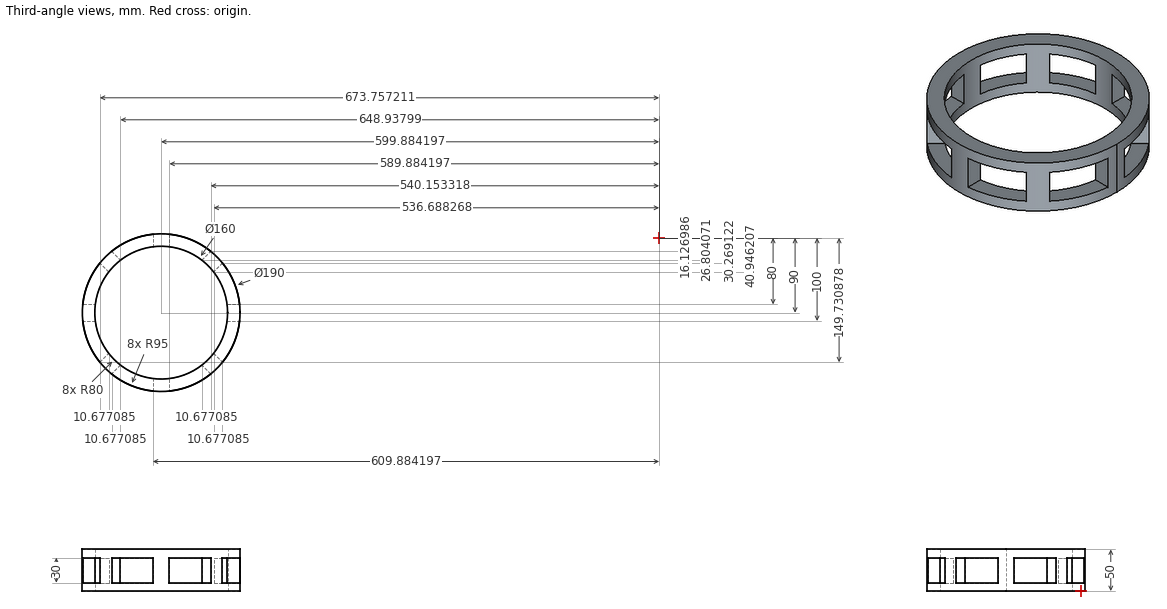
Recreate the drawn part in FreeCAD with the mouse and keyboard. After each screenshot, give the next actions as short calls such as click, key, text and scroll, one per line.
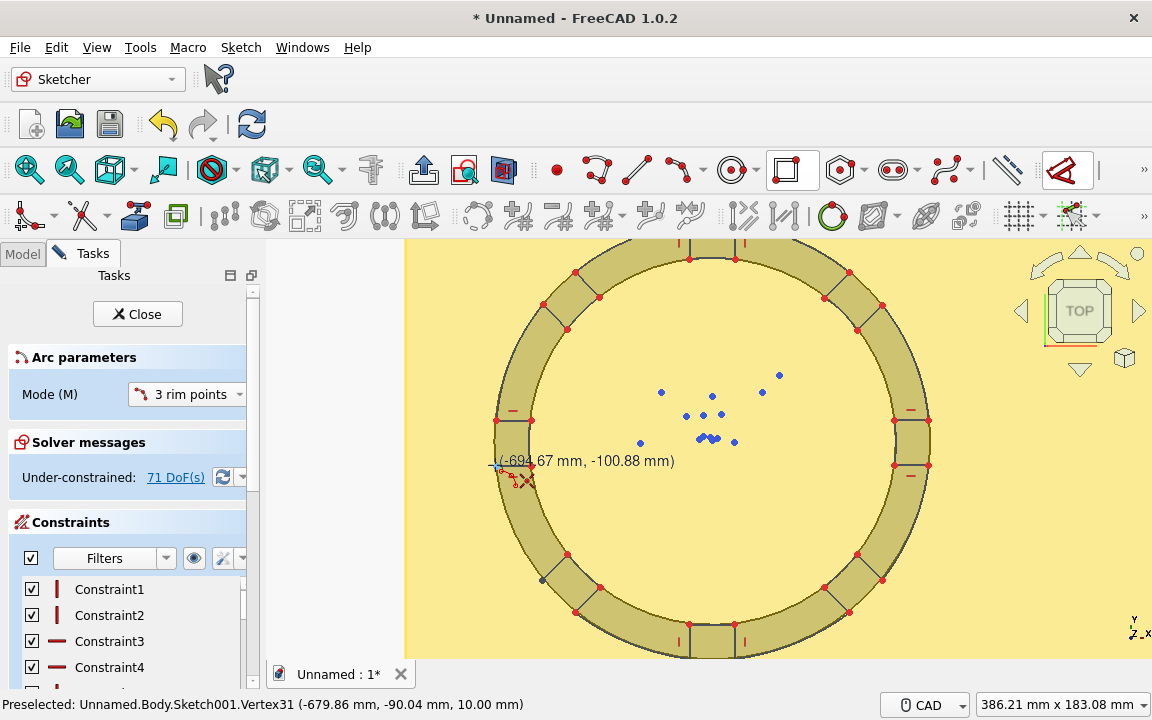
click(496, 466)
click(542, 580)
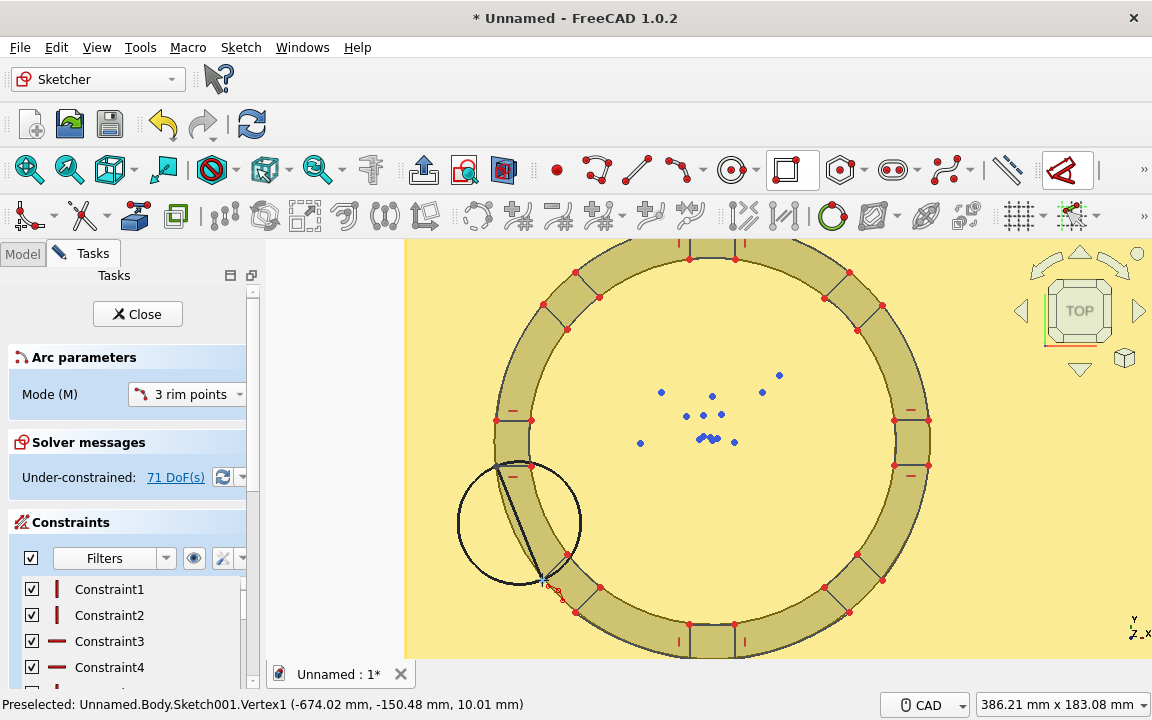
scroll(511, 525, up, 3)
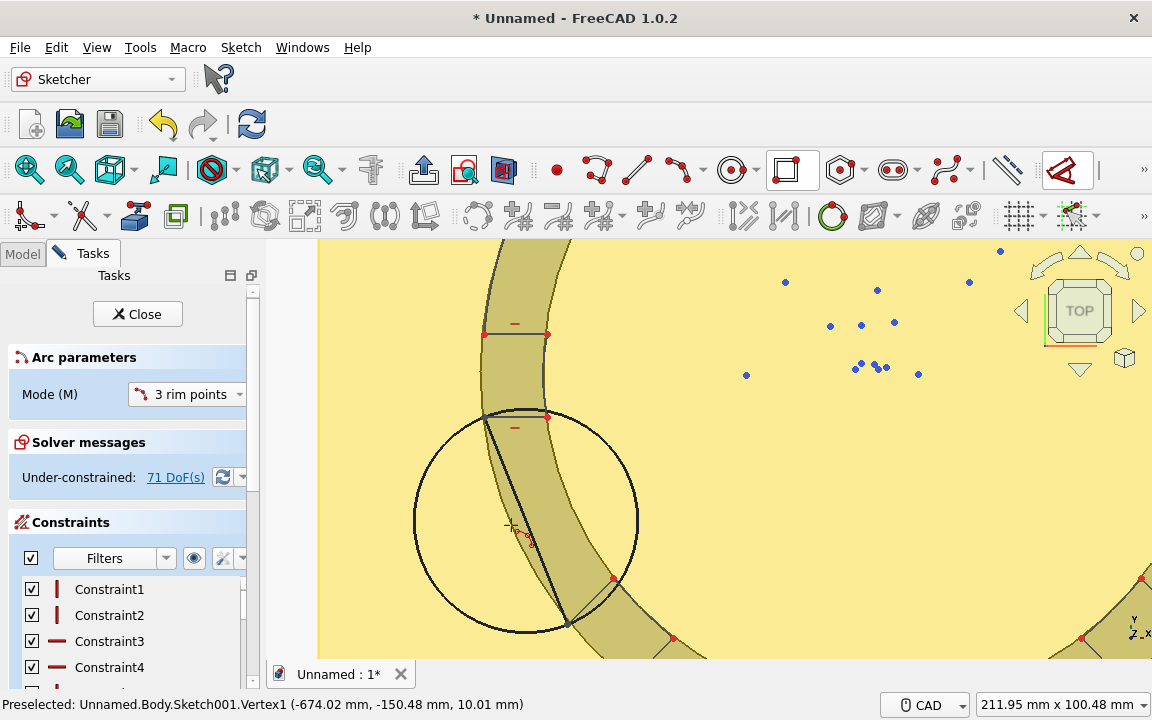
click(511, 524)
key(Escape)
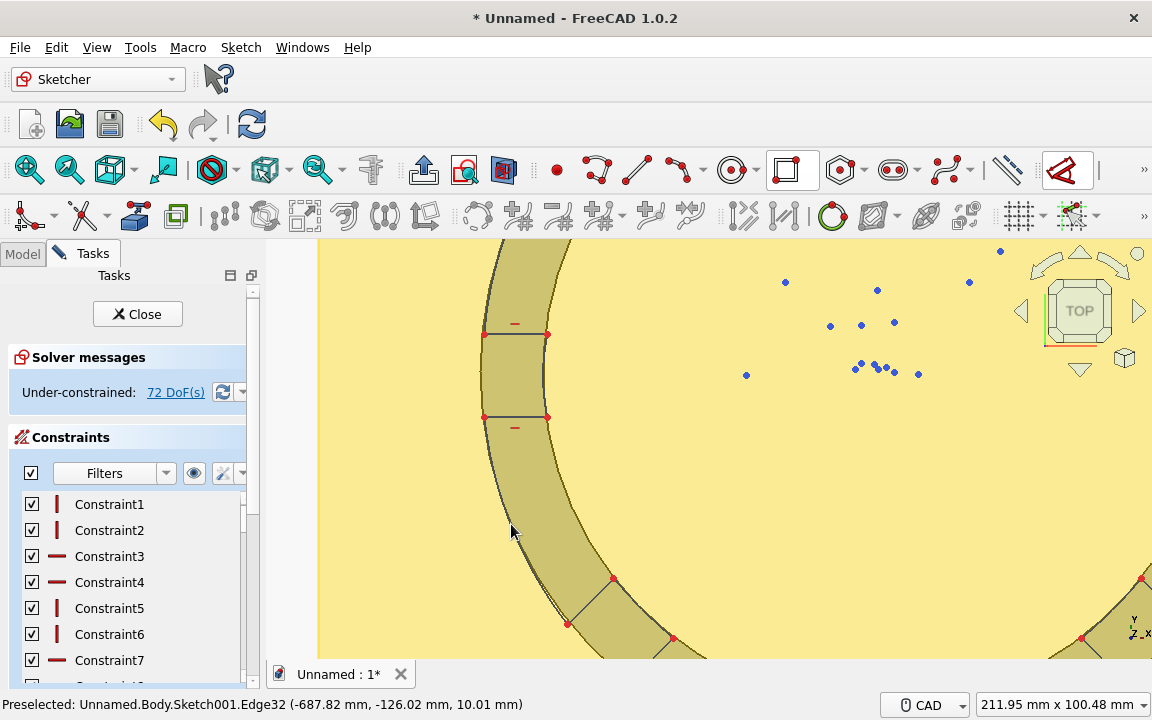
click(631, 598)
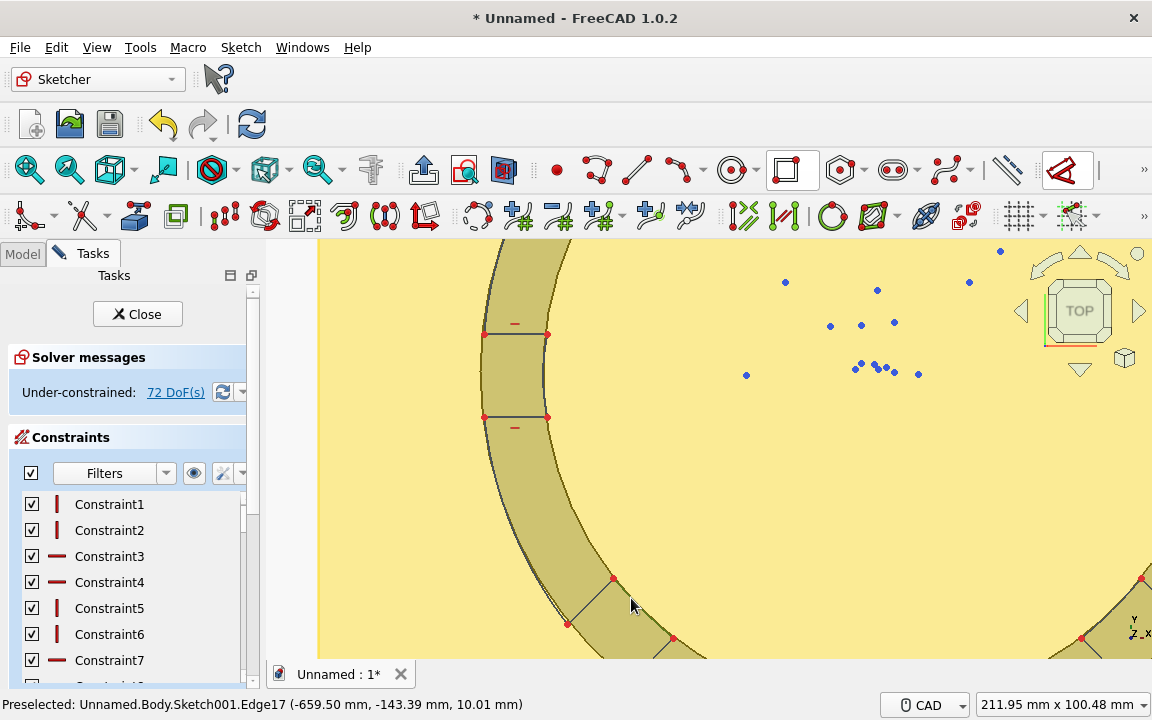
scroll(538, 482, down, 6)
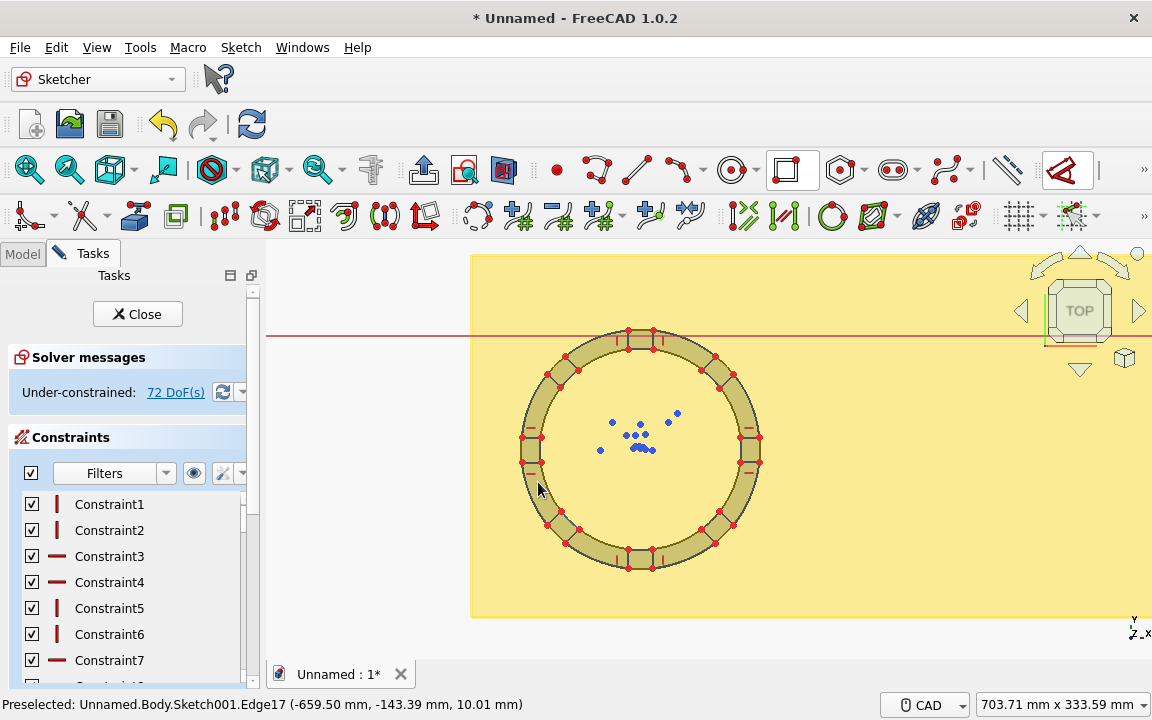
click(583, 554)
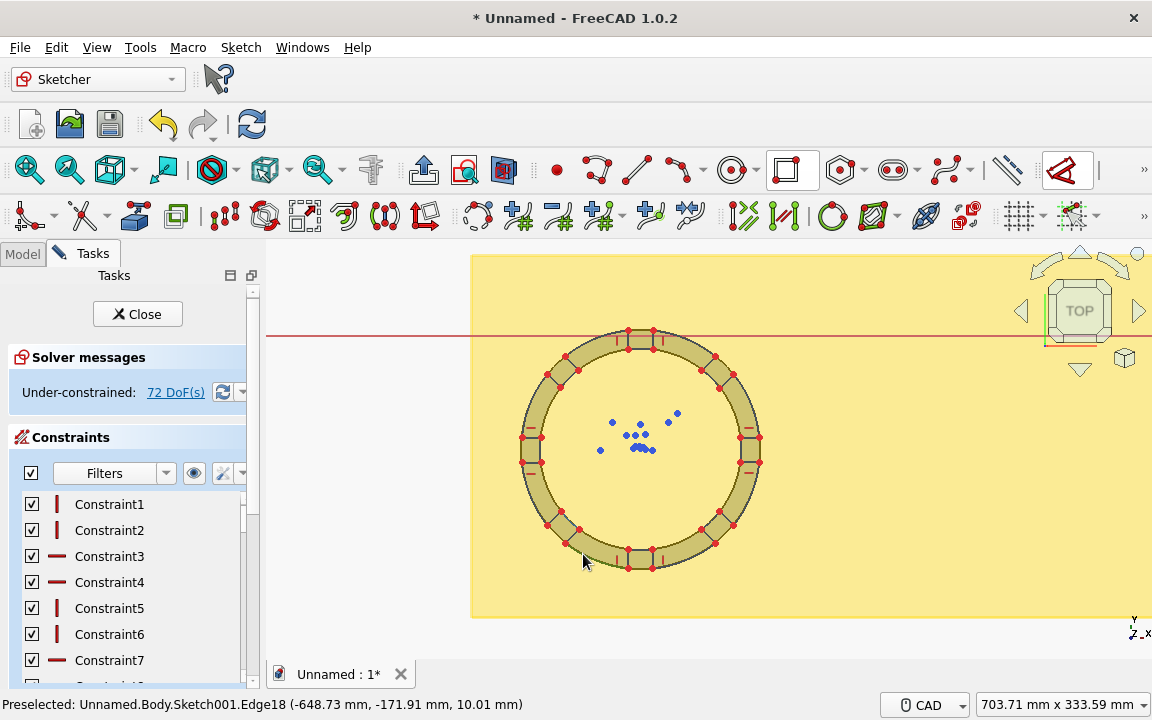
key(c)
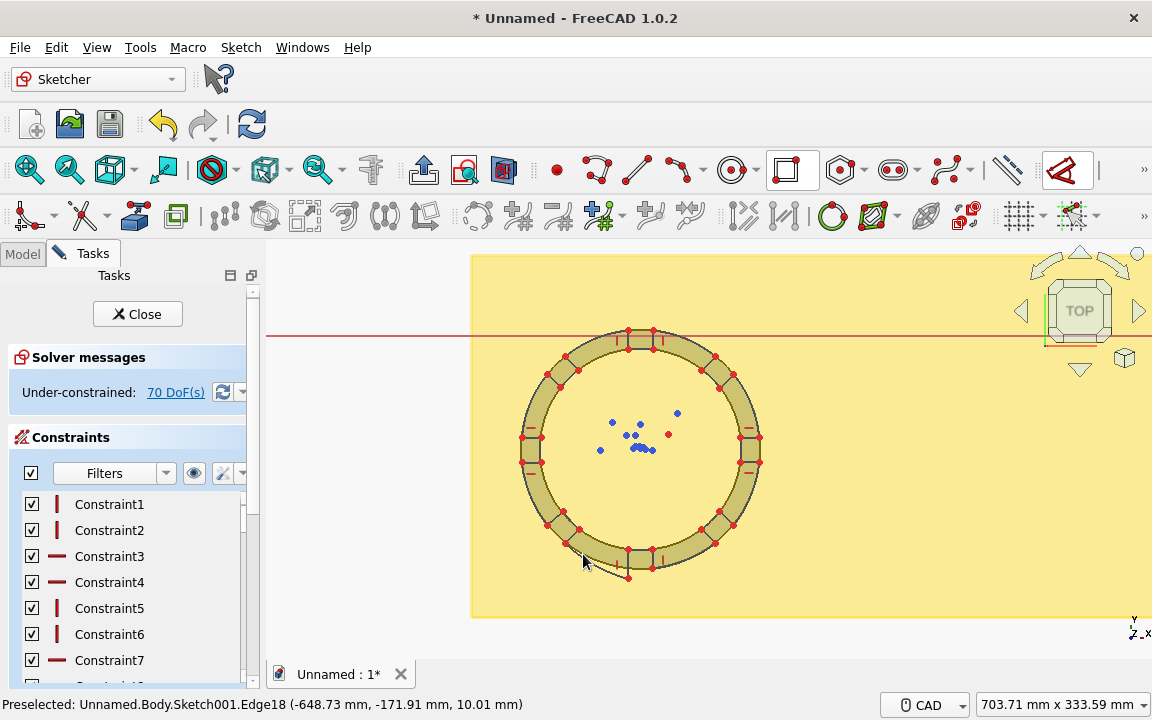
click(571, 521)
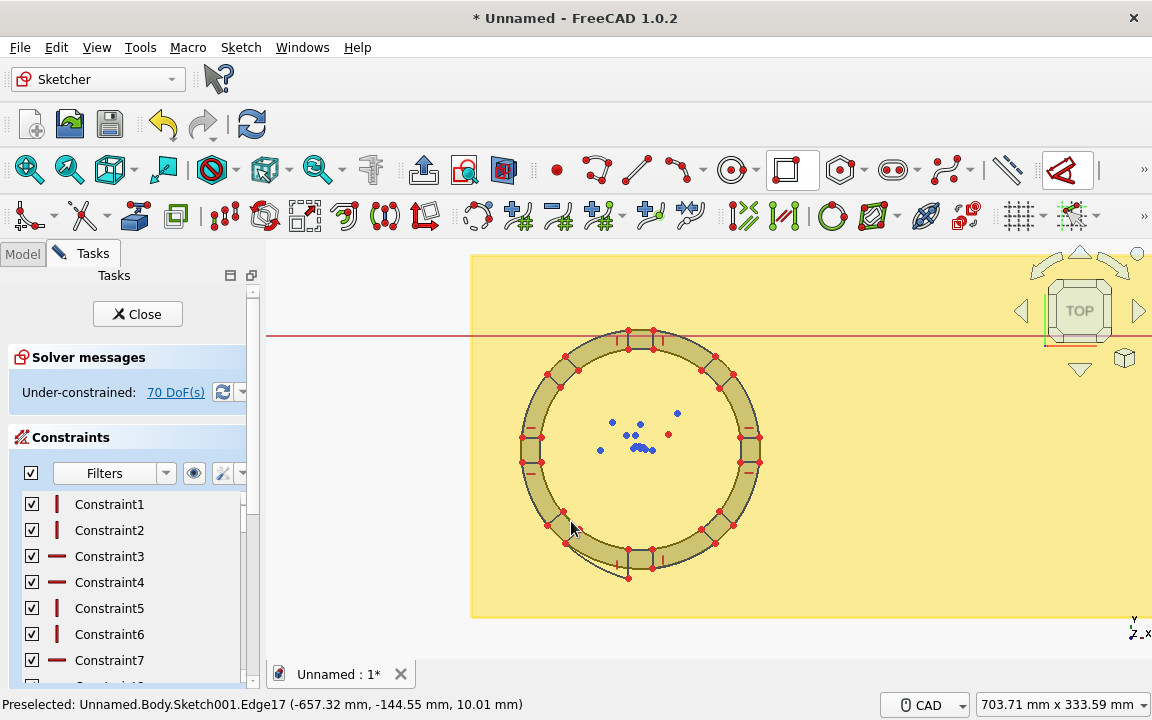
click(640, 550)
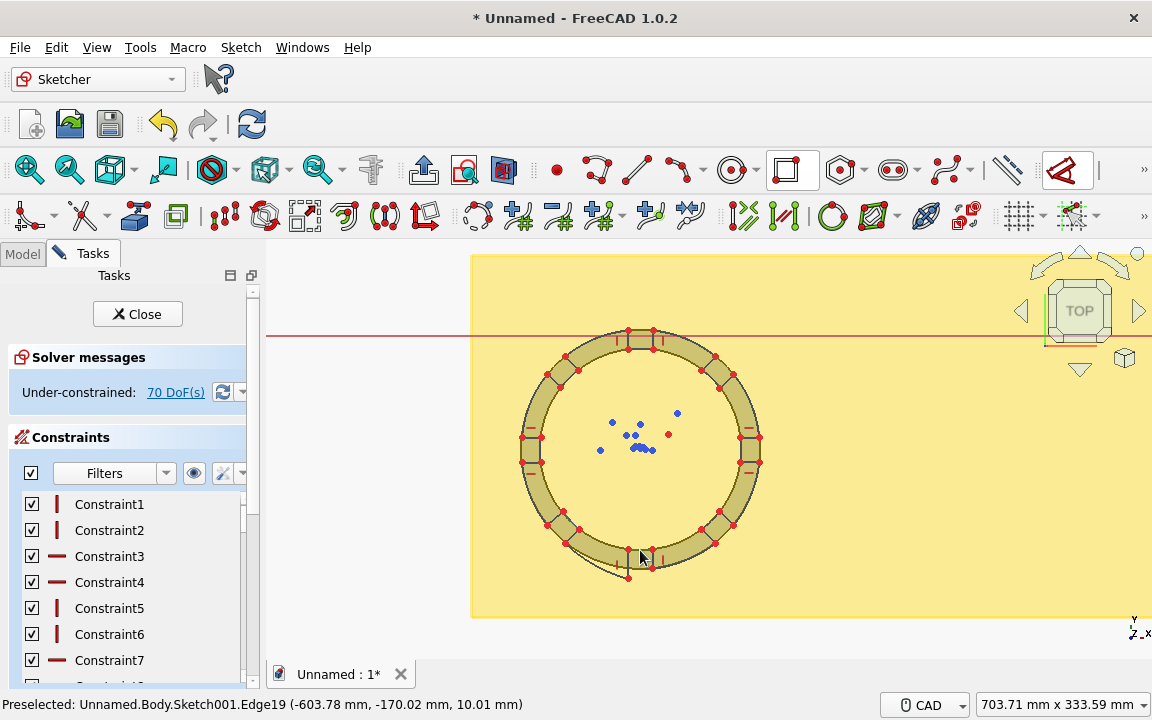
key(c)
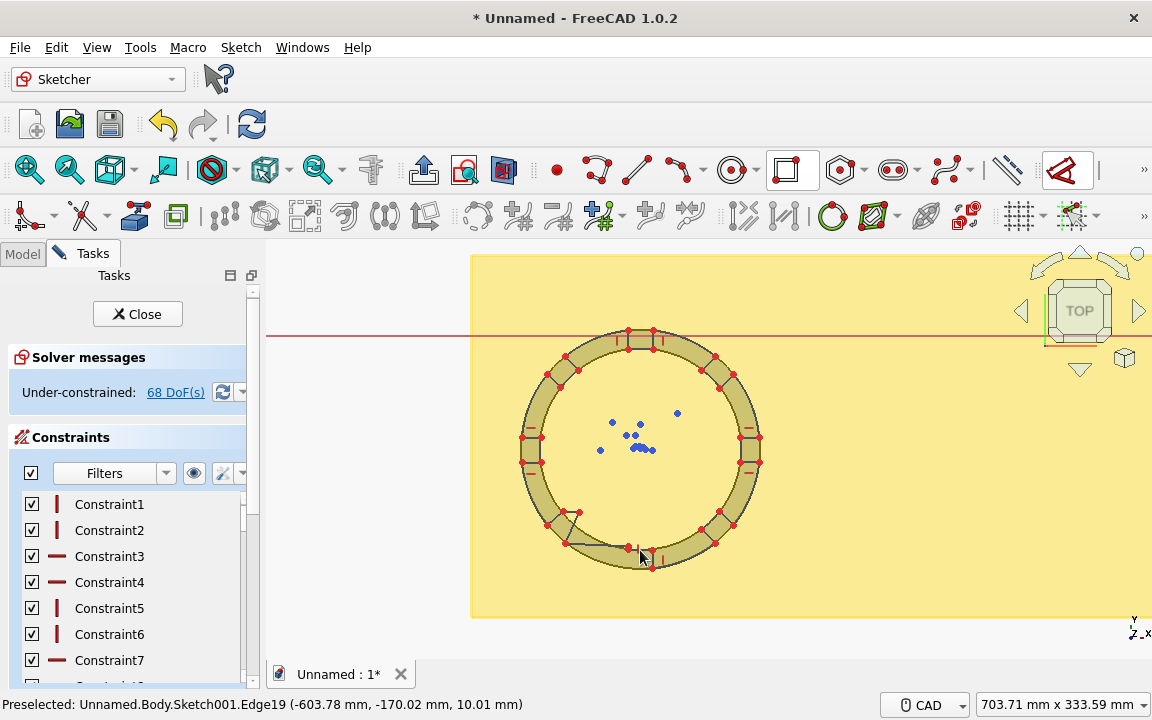
scroll(571, 512, up, 4)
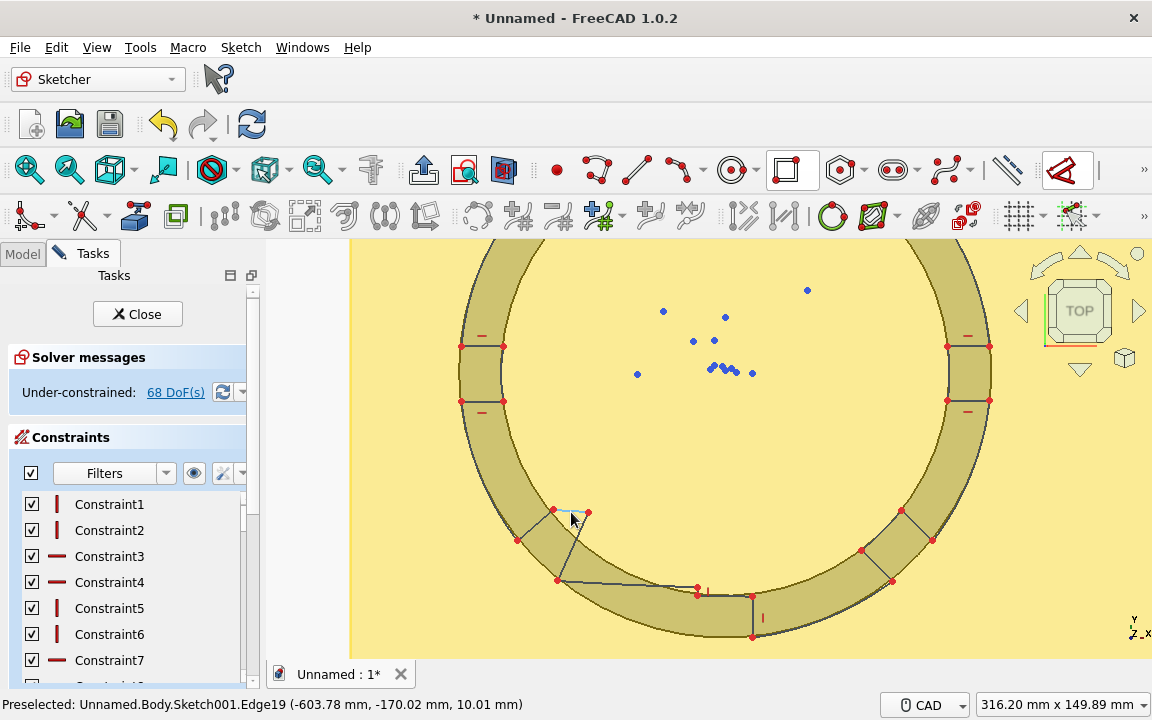
click(571, 511)